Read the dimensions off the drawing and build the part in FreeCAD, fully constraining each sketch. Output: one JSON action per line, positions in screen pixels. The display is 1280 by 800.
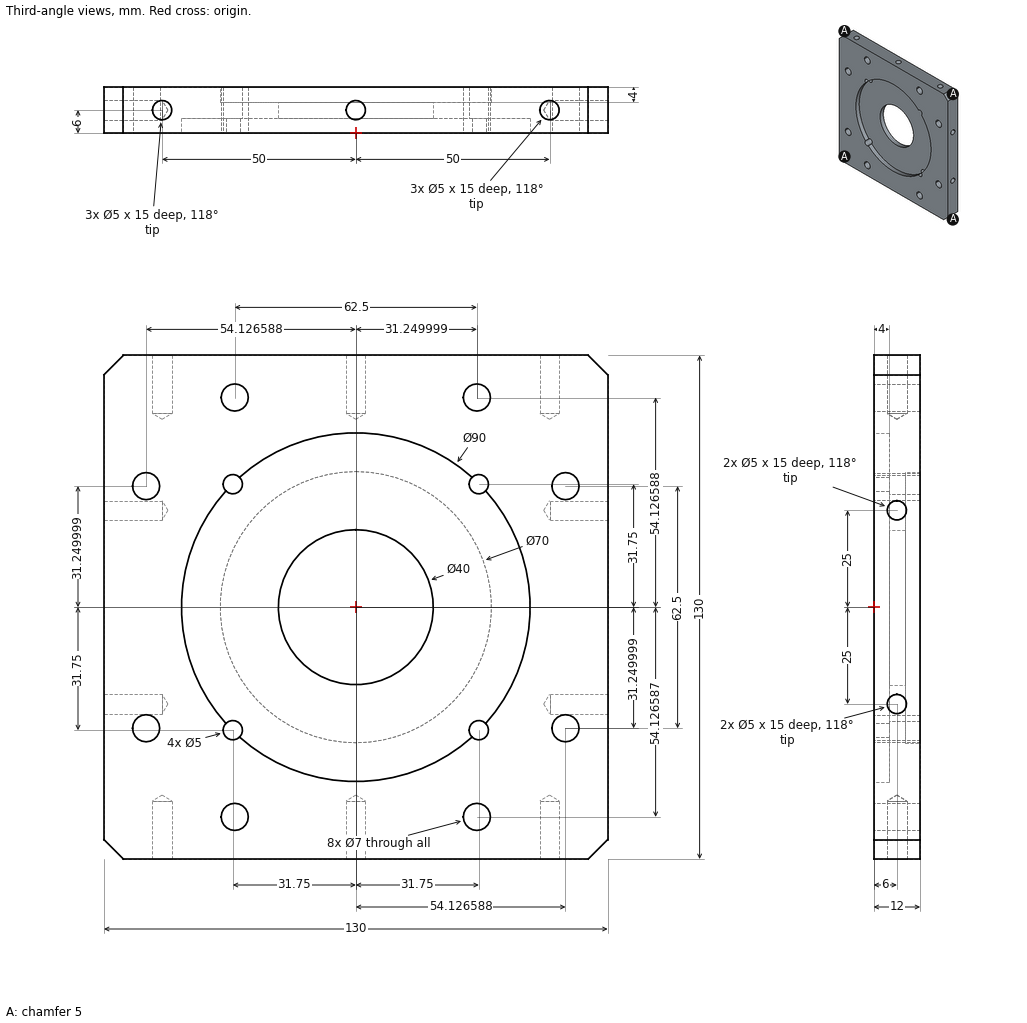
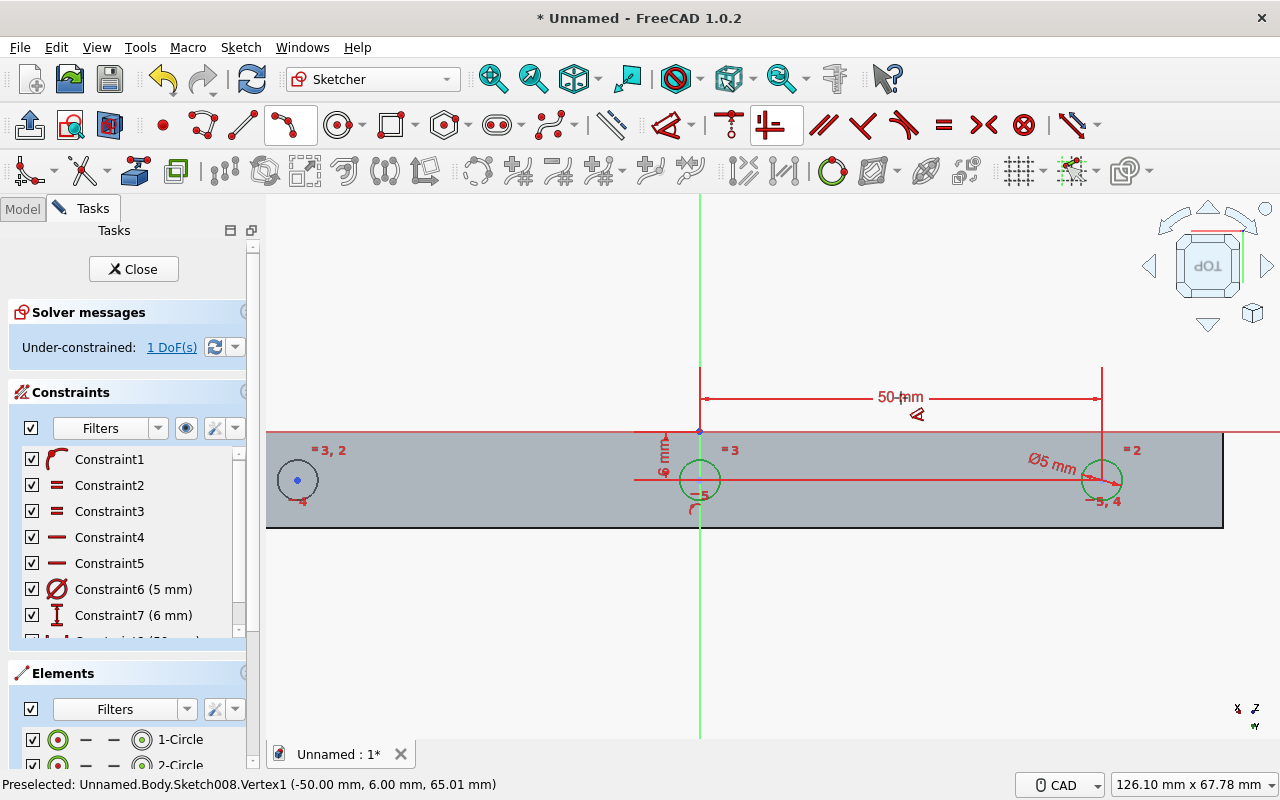
{"action": "left_click", "coordinate": [298, 480]}
{"action": "left_click", "coordinate": [499, 398]}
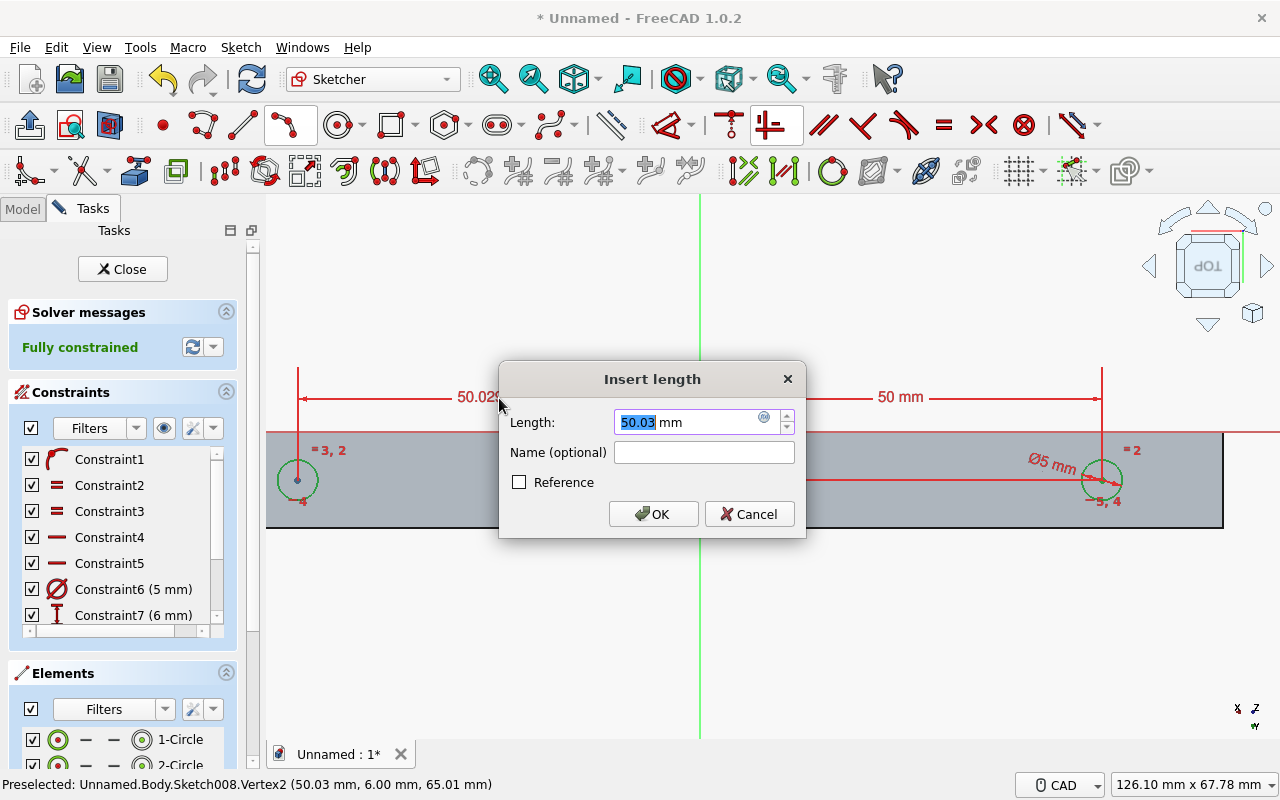
{"action": "type", "text": "50"}
{"action": "key", "text": "Return"}
{"action": "key", "text": "Escape"}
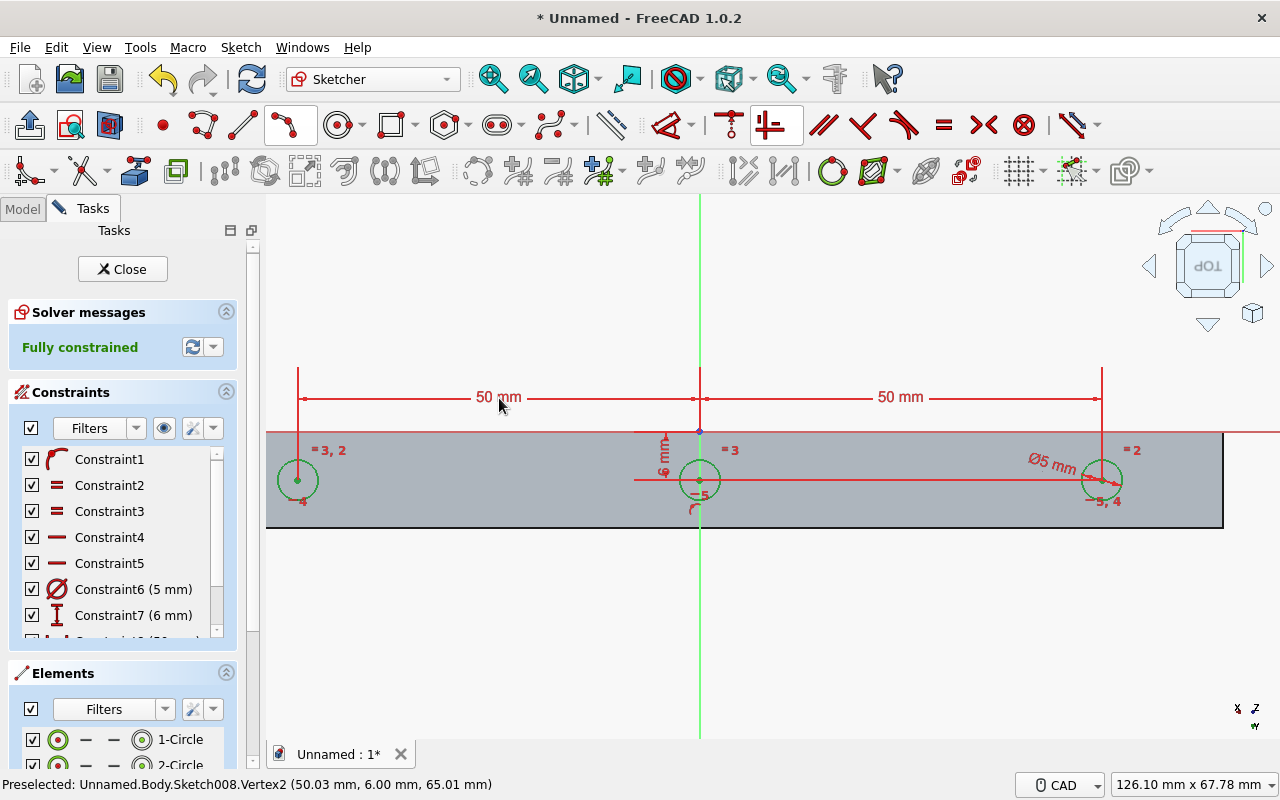
{"action": "left_click", "coordinate": [123, 269]}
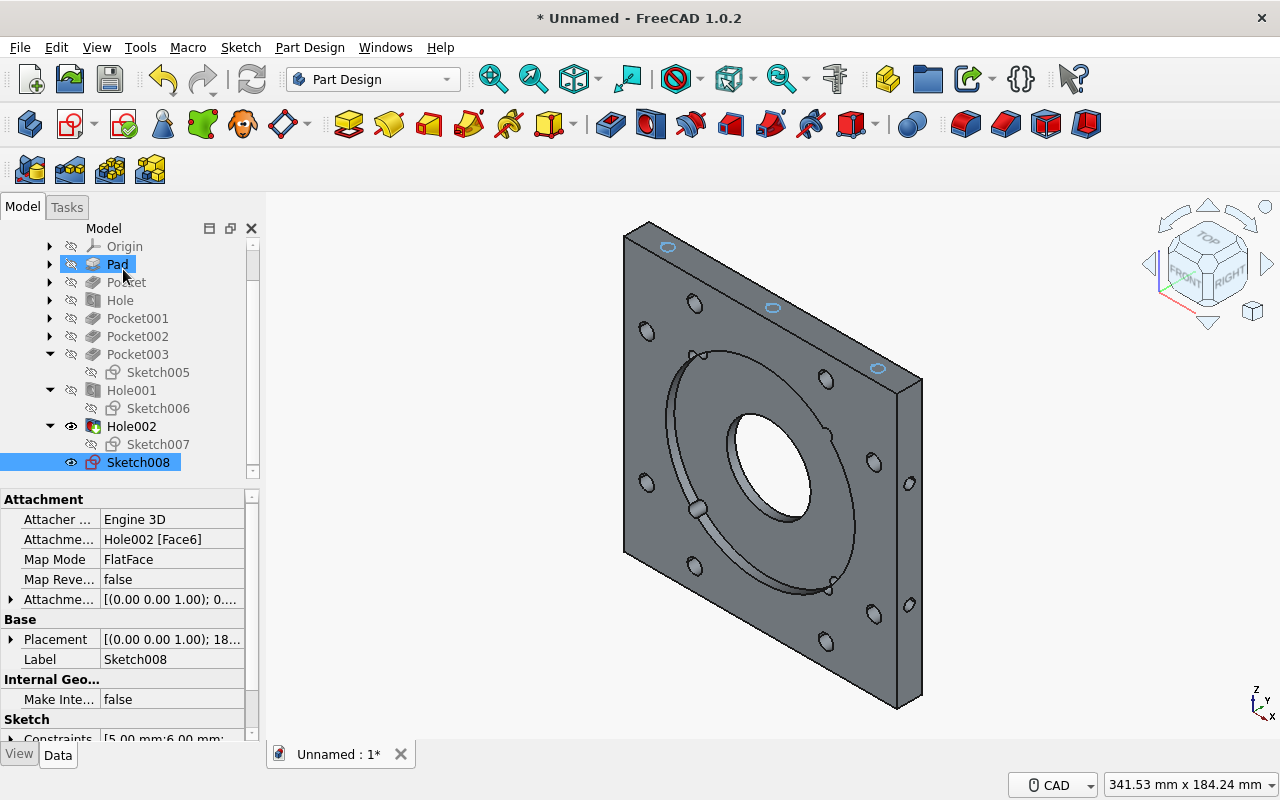
{"action": "left_click", "coordinate": [652, 124]}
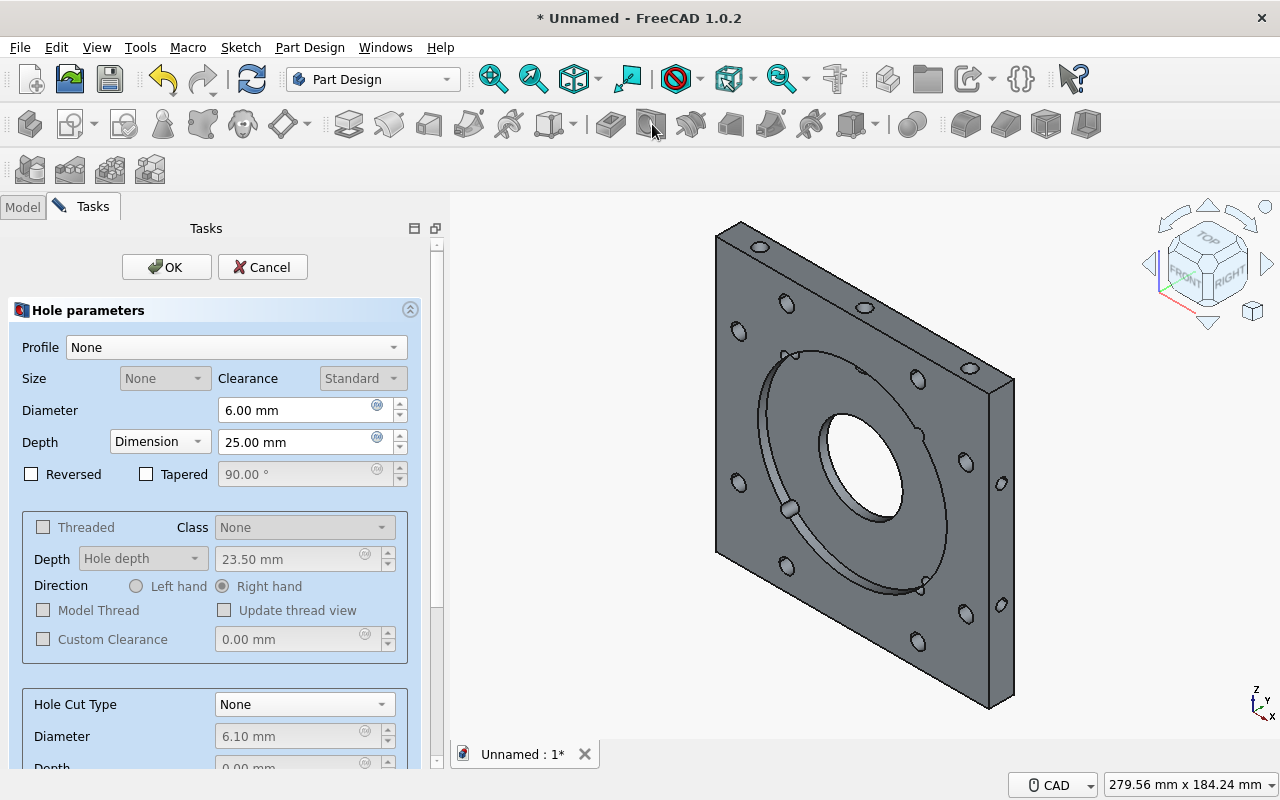
{"action": "triple_click", "coordinate": [305, 410]}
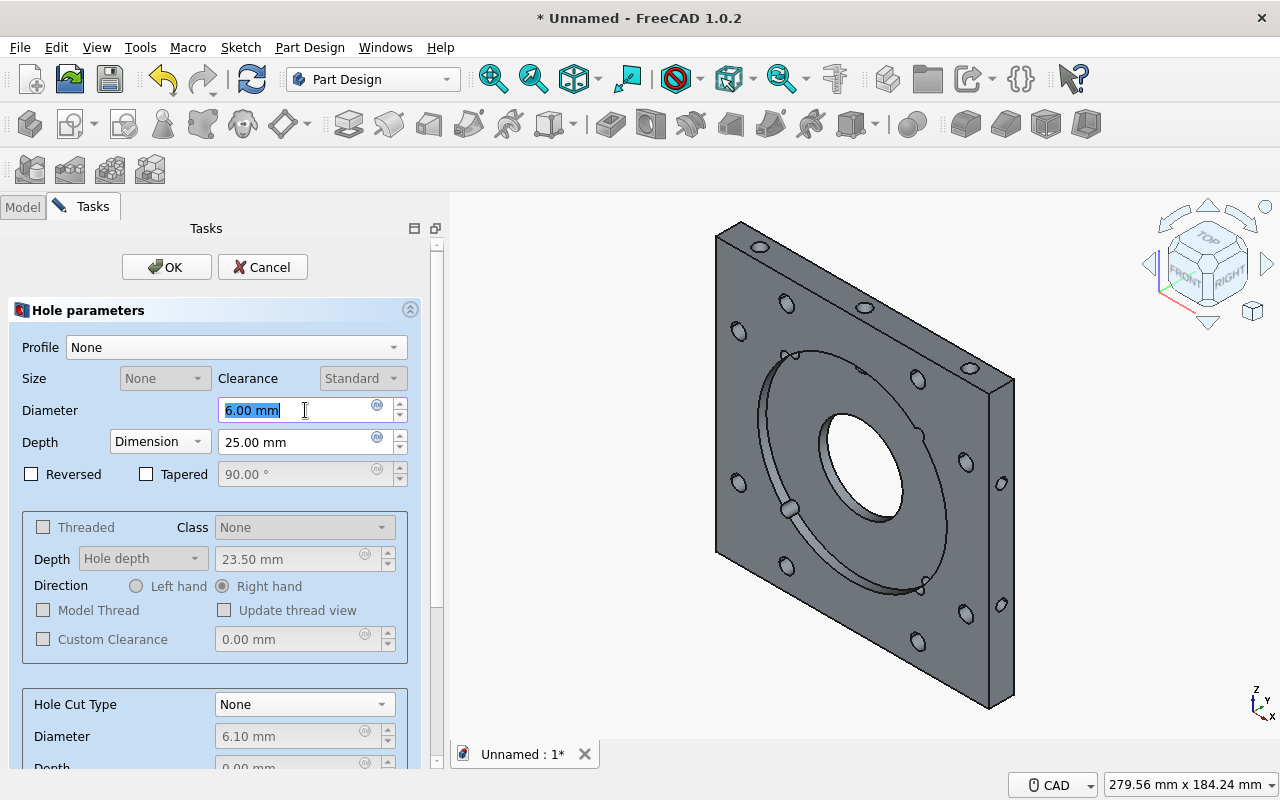
{"action": "type", "text": "5"}
{"action": "key", "text": "Tab"}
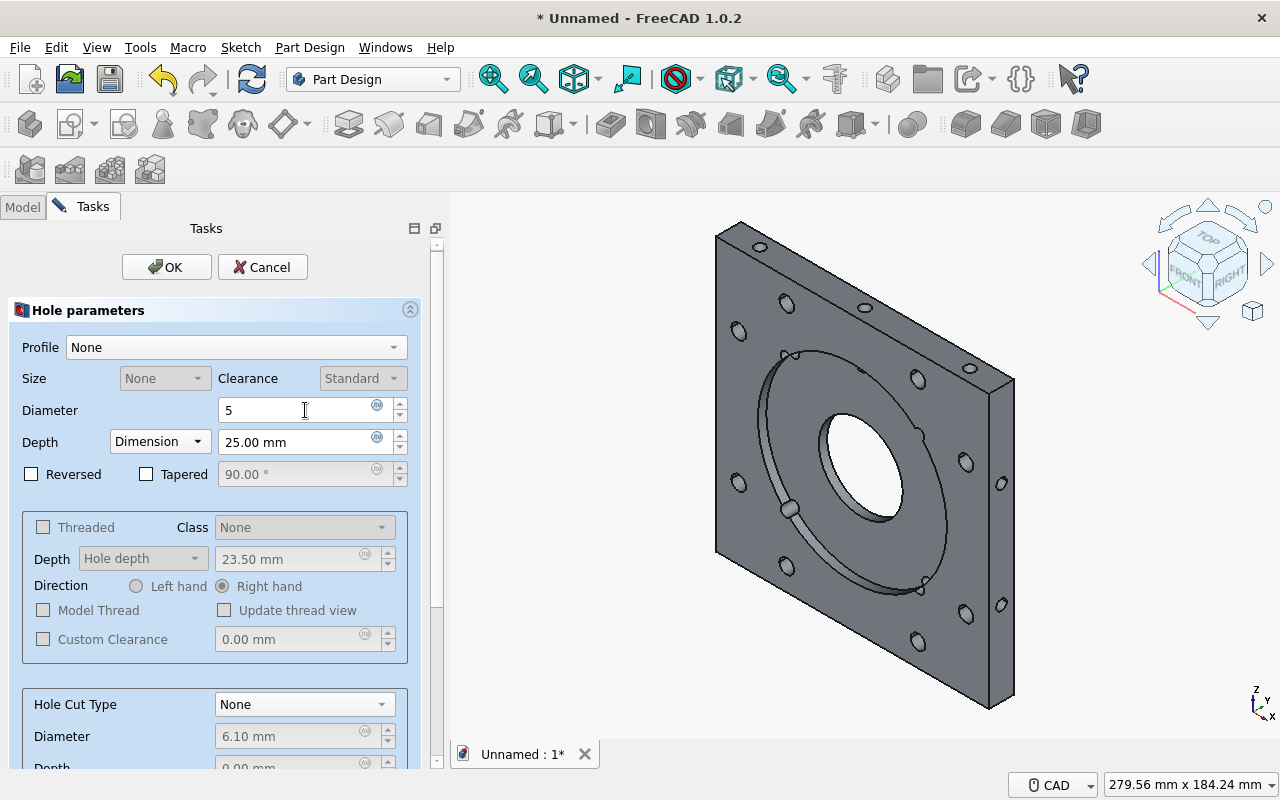
{"action": "triple_click", "coordinate": [305, 442]}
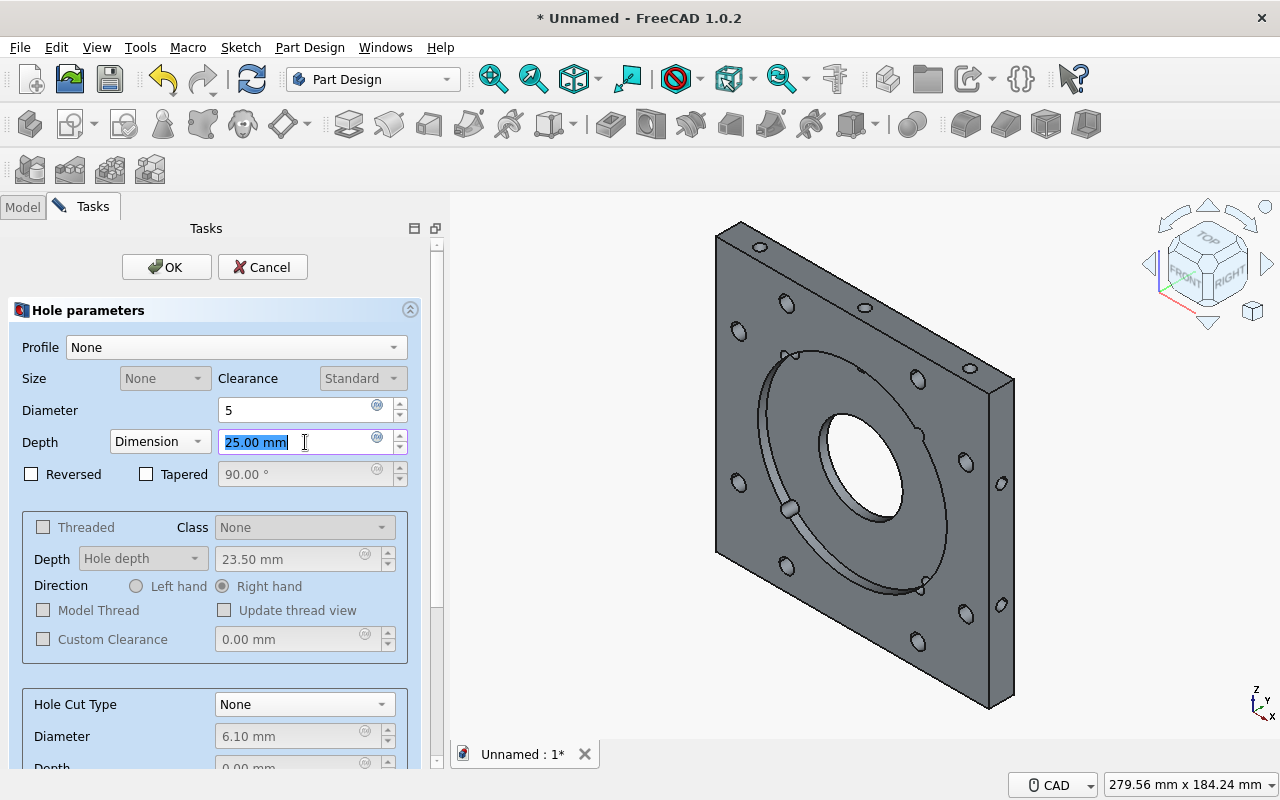
{"action": "type", "text": "15"}
{"action": "key", "text": "Tab"}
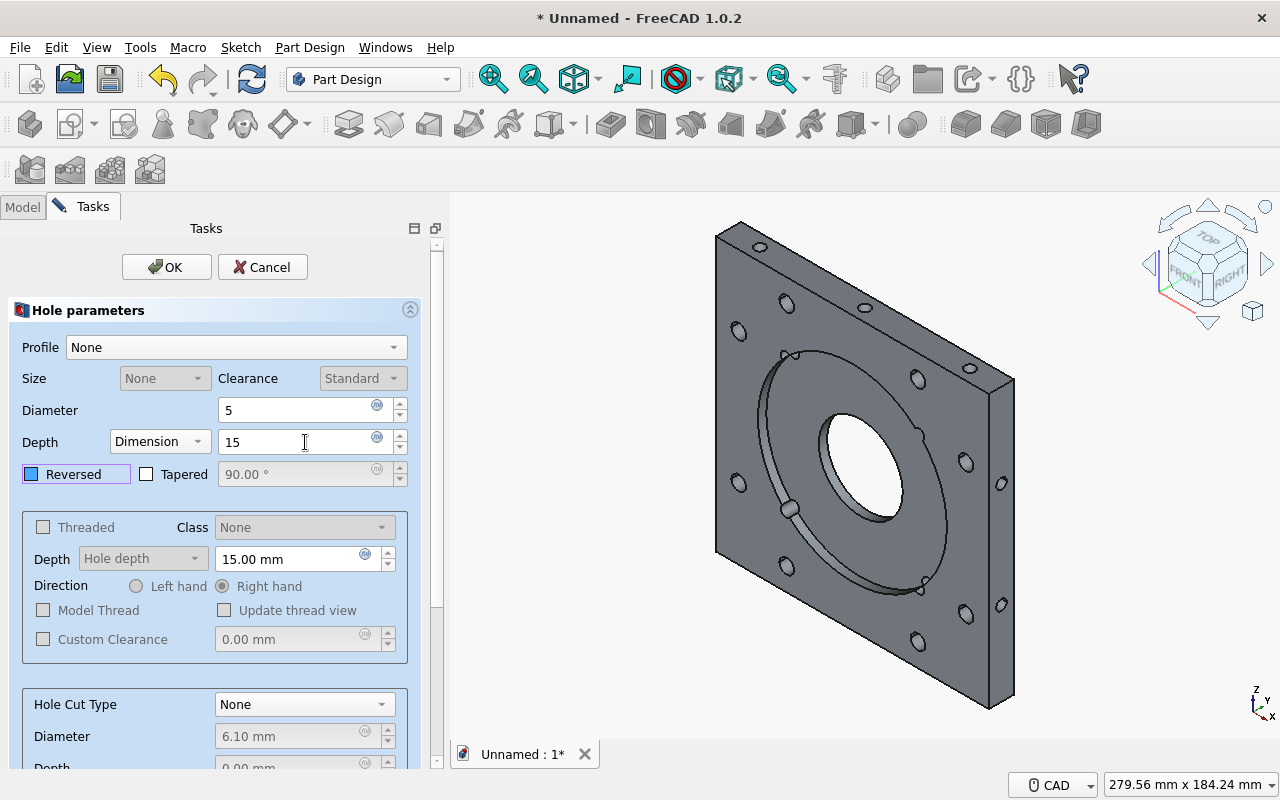
{"action": "left_click", "coordinate": [167, 267]}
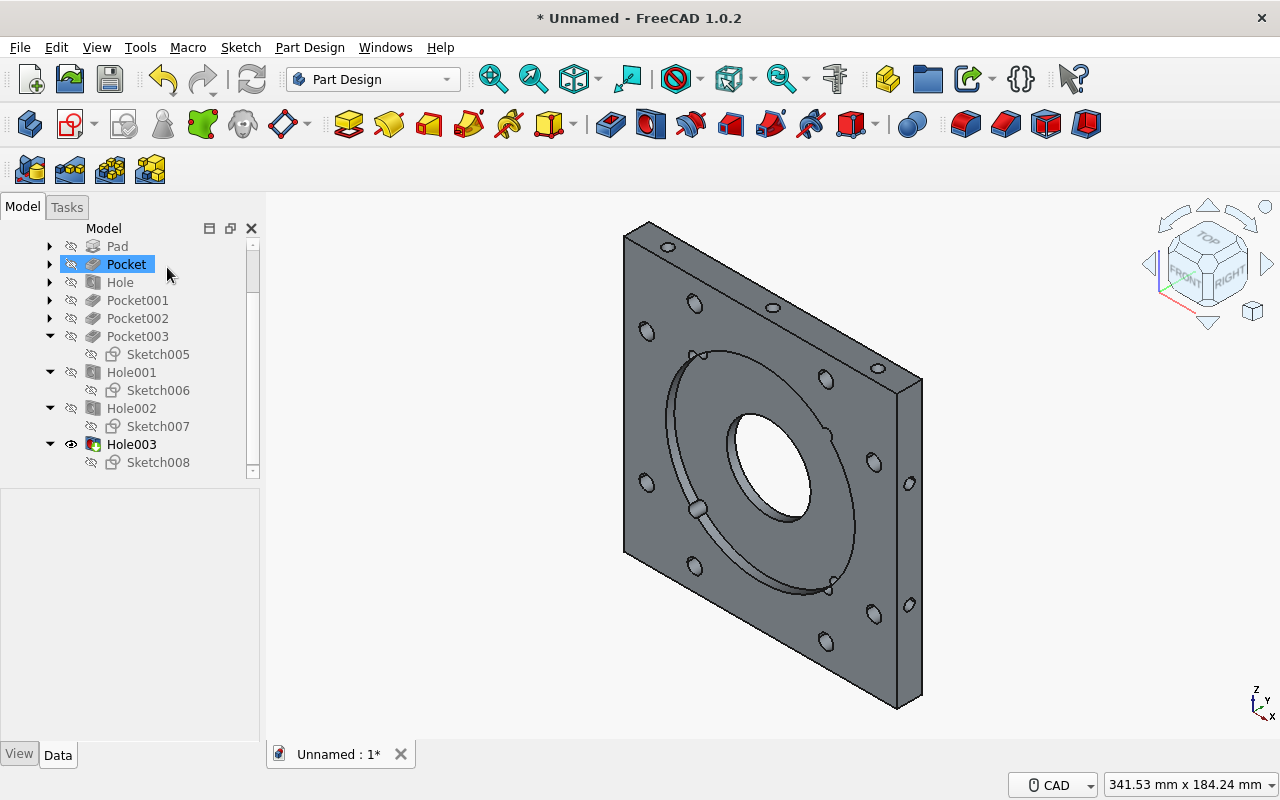
{"action": "key", "text": "5"}